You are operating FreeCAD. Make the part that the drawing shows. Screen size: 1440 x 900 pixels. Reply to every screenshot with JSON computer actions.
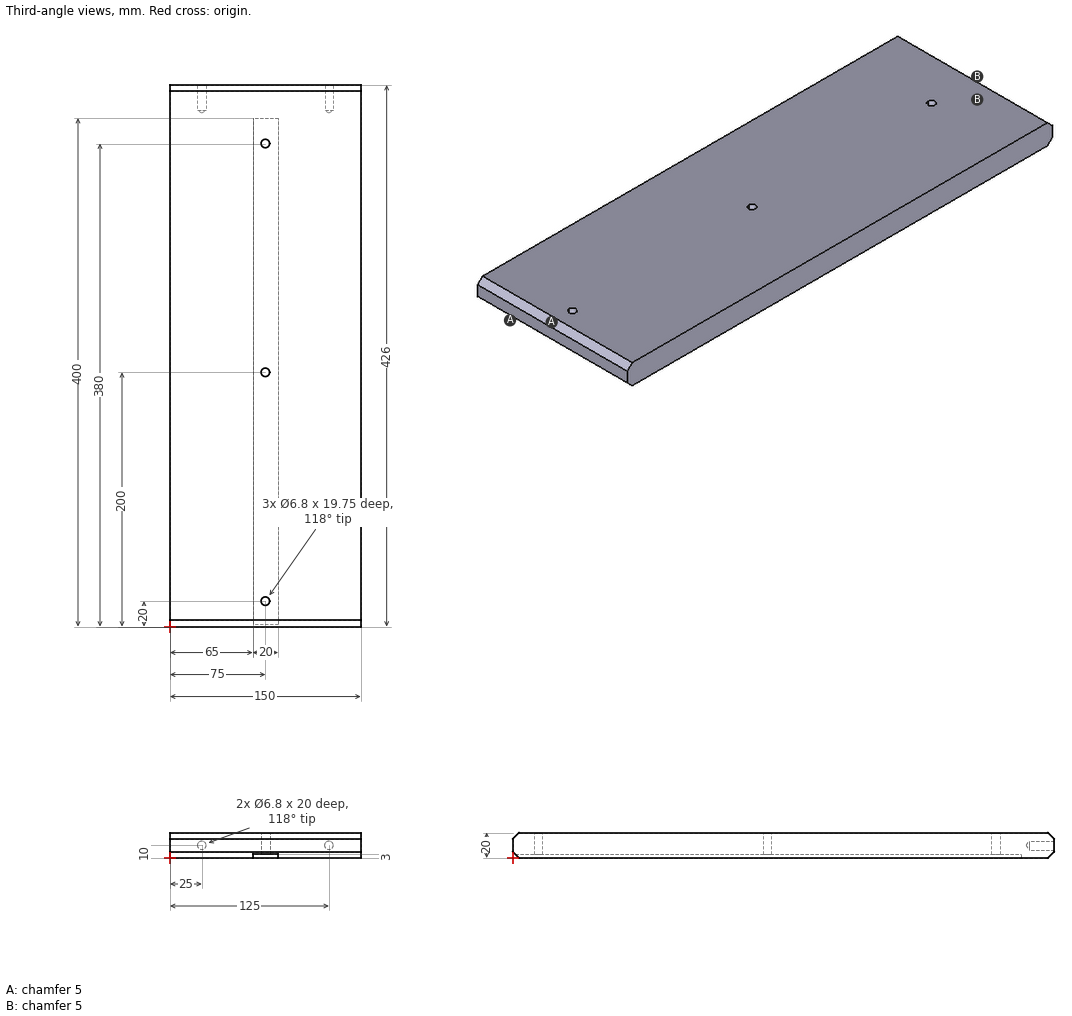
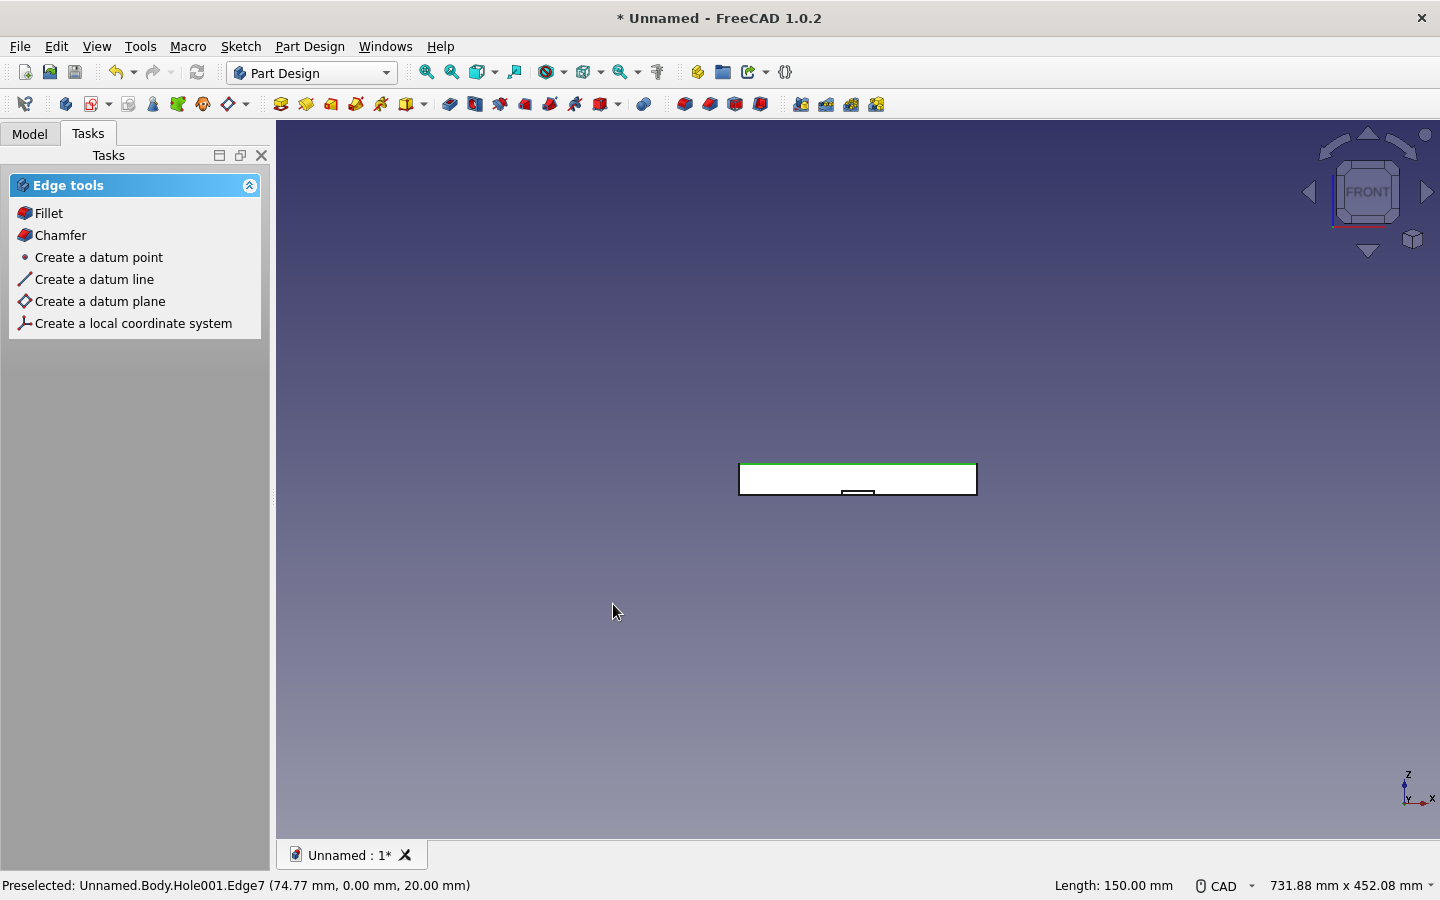
{"action": "key", "text": "v f"}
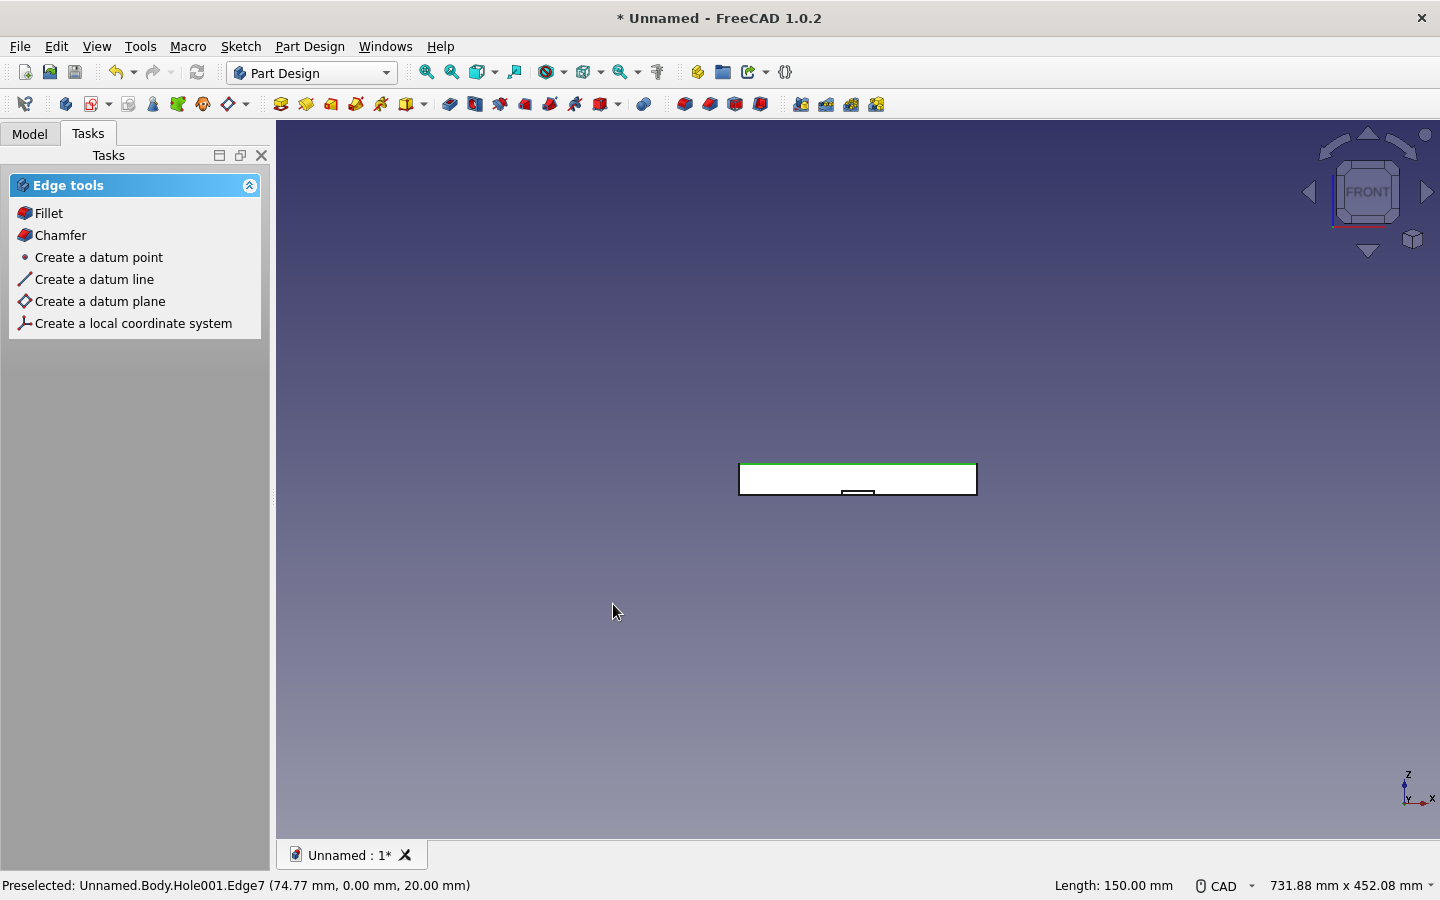
{"action": "left_click", "coordinate": [790, 494], "text": "ctrl"}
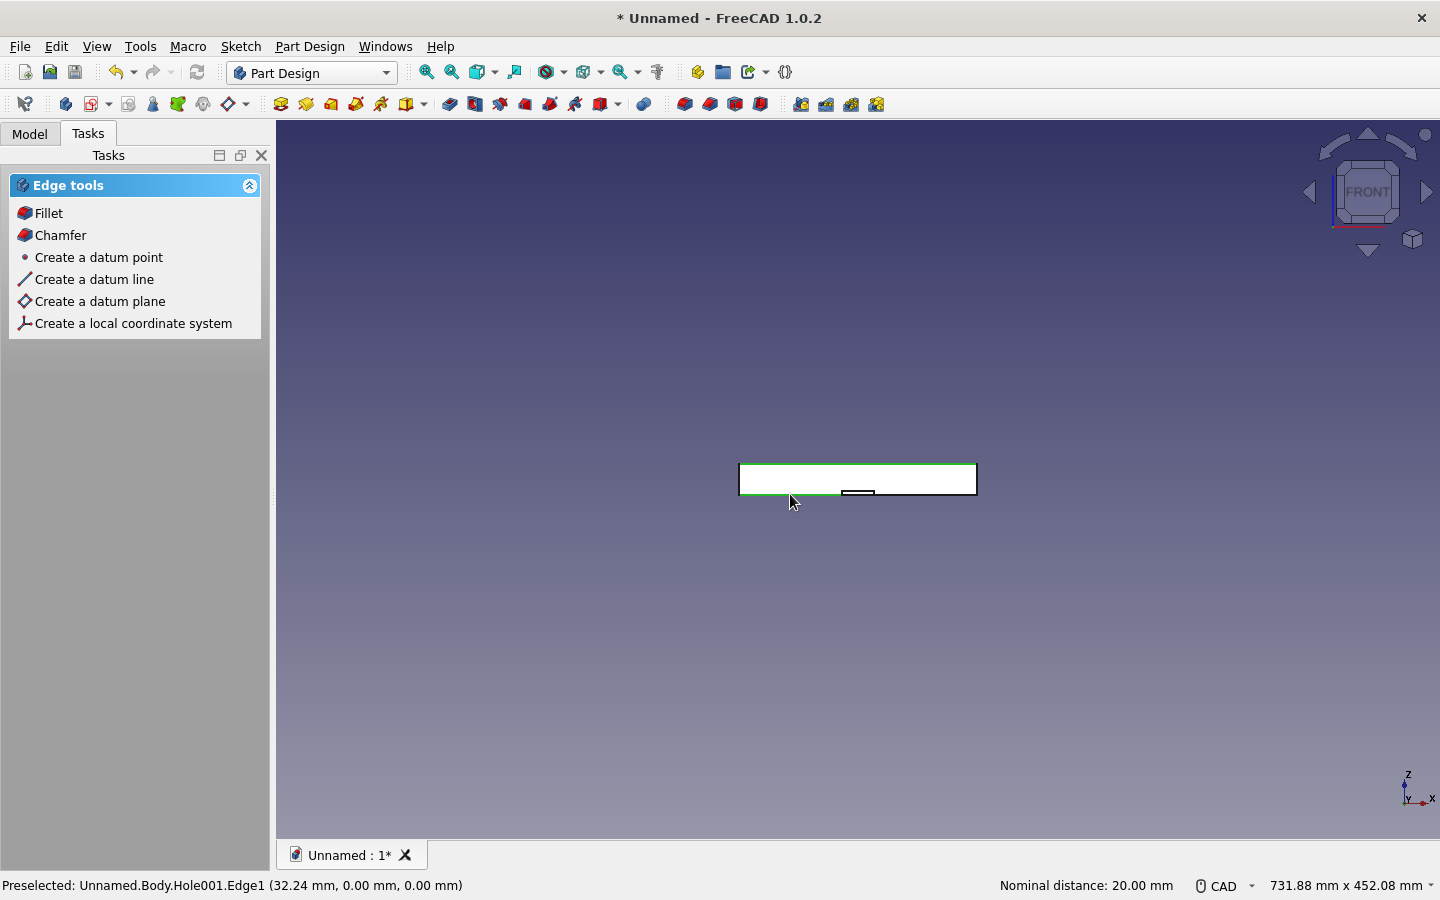
{"action": "left_click", "coordinate": [710, 104]}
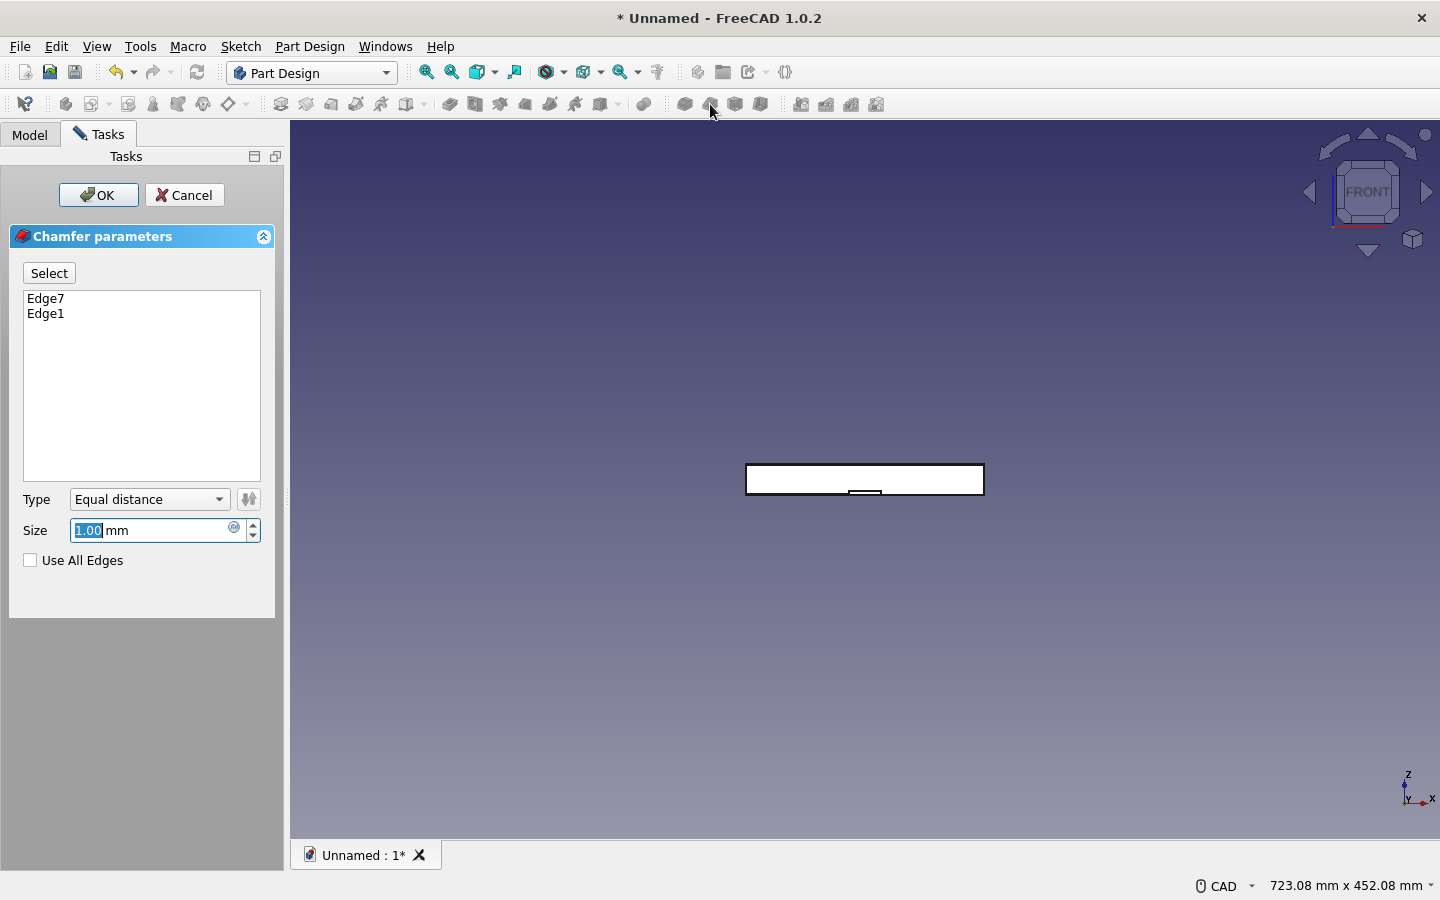
{"action": "type", "text": "5"}
{"action": "key", "text": "Tab"}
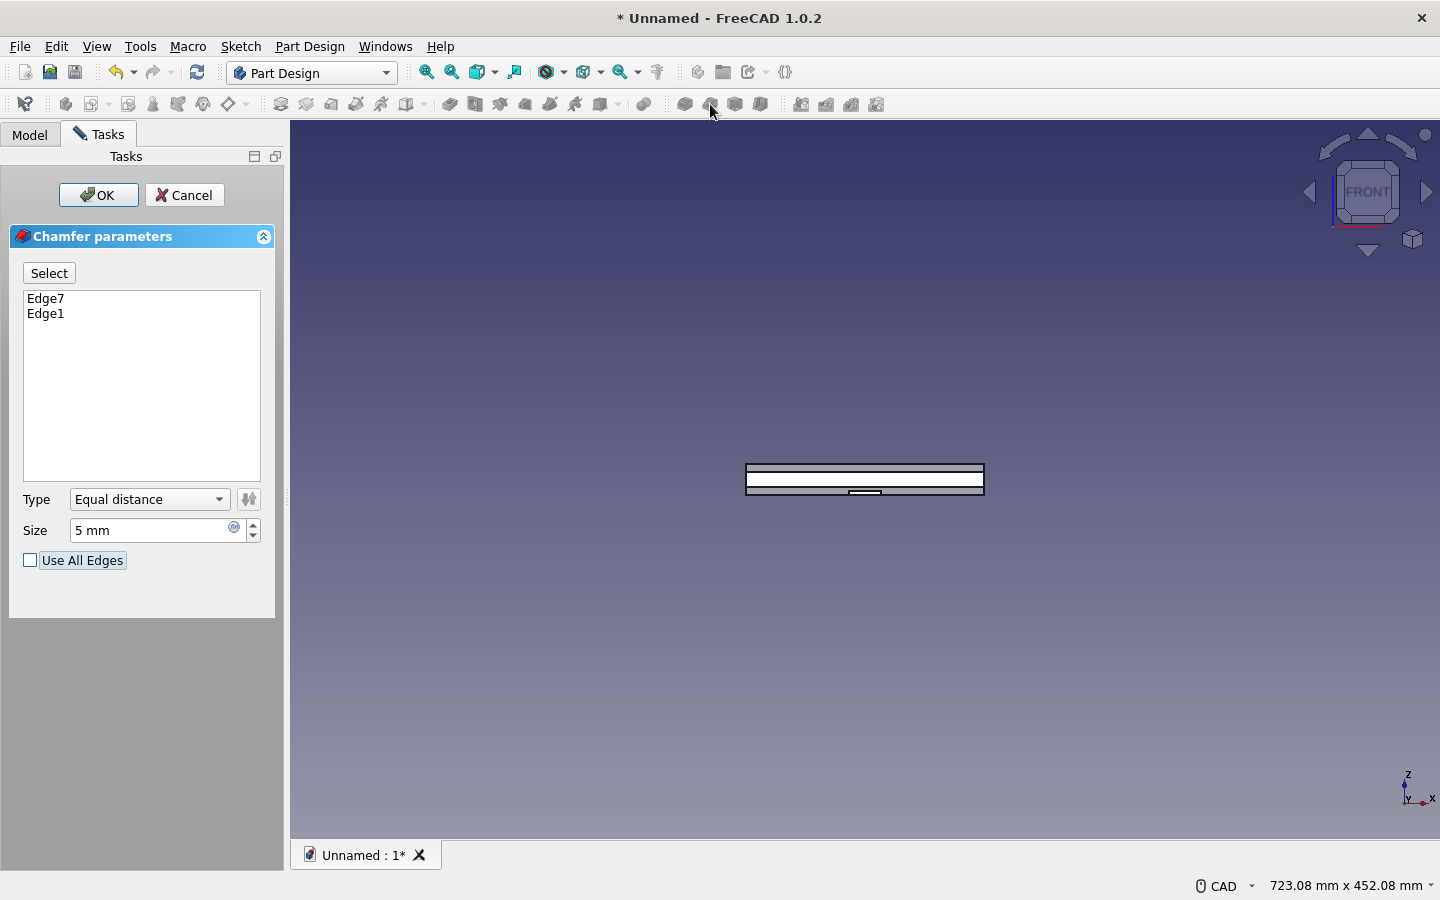
{"action": "left_click", "coordinate": [99, 195]}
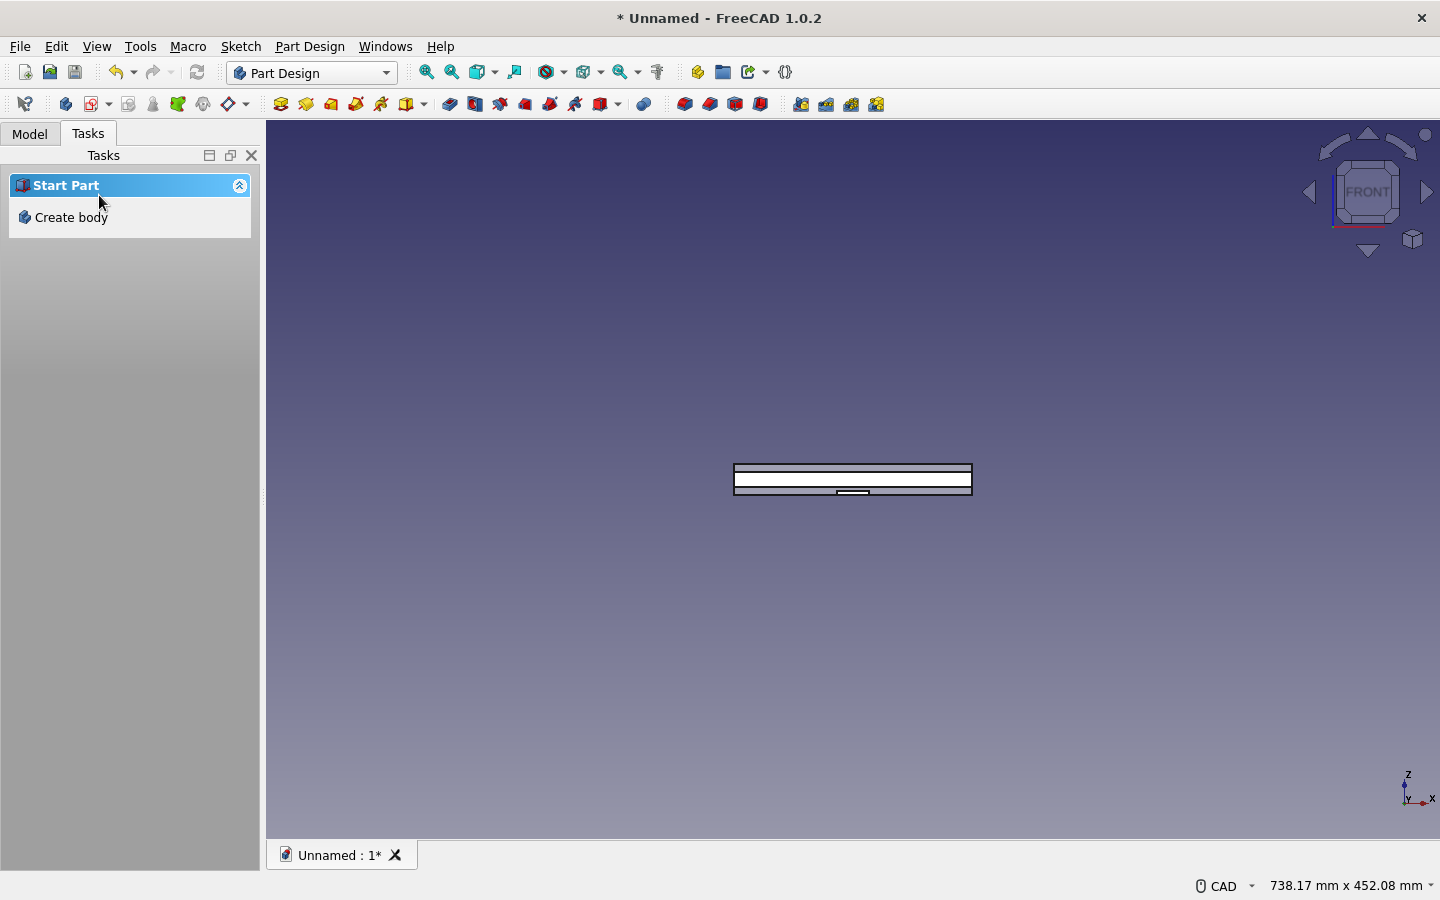
{"action": "left_click", "coordinate": [427, 72]}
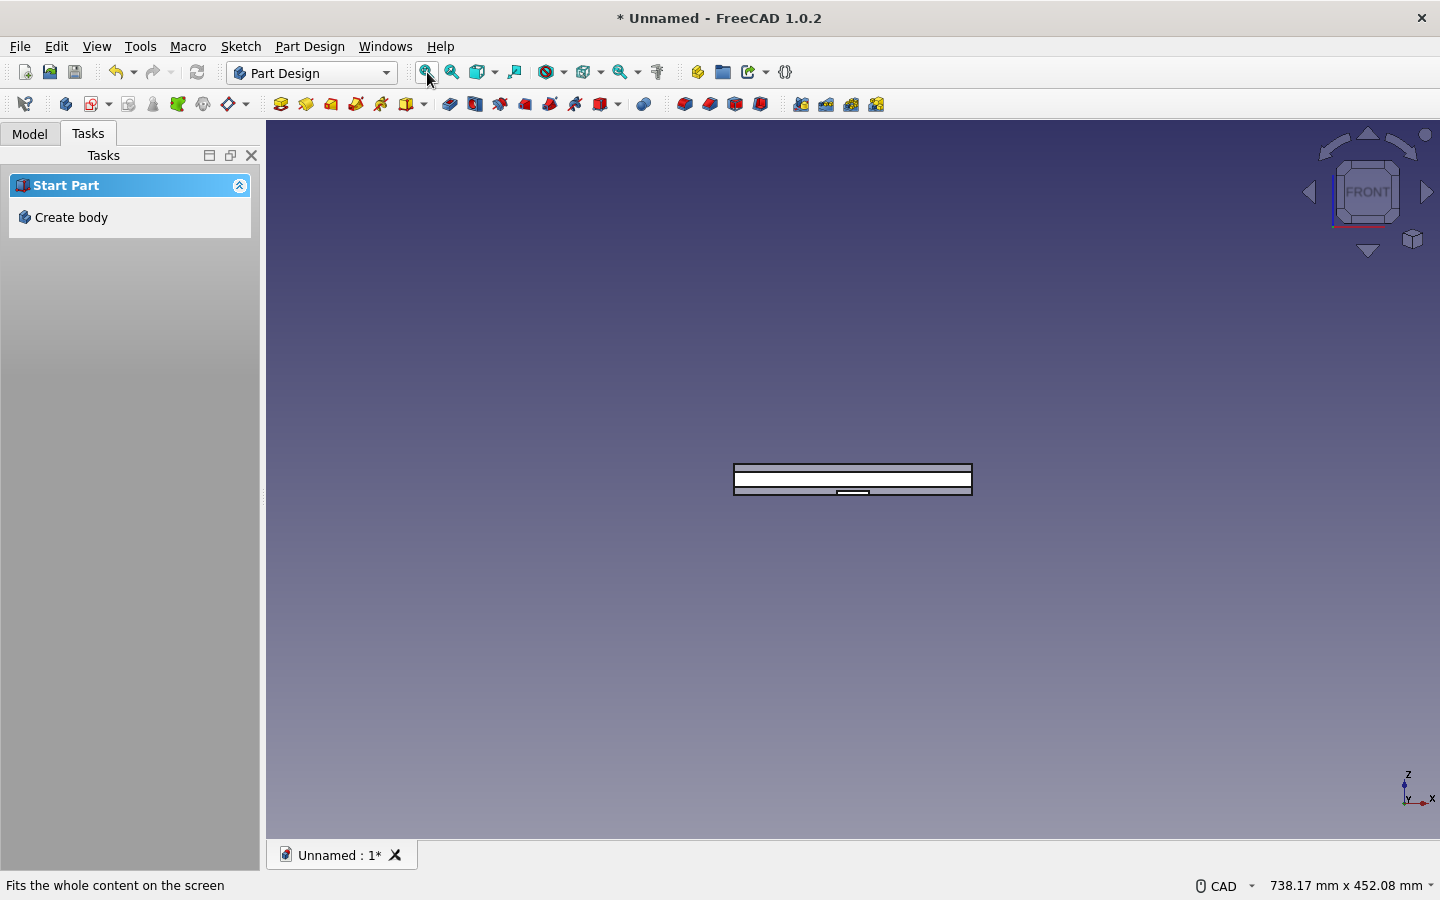
{"action": "key", "text": "0"}